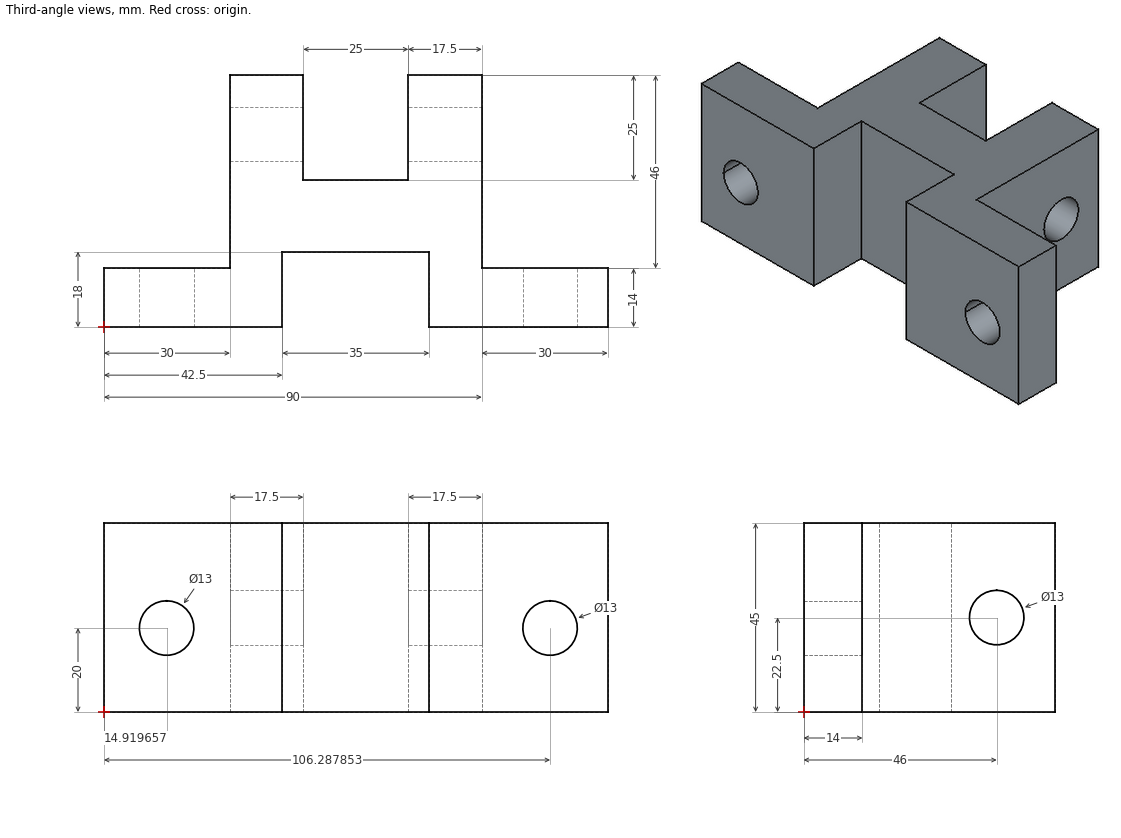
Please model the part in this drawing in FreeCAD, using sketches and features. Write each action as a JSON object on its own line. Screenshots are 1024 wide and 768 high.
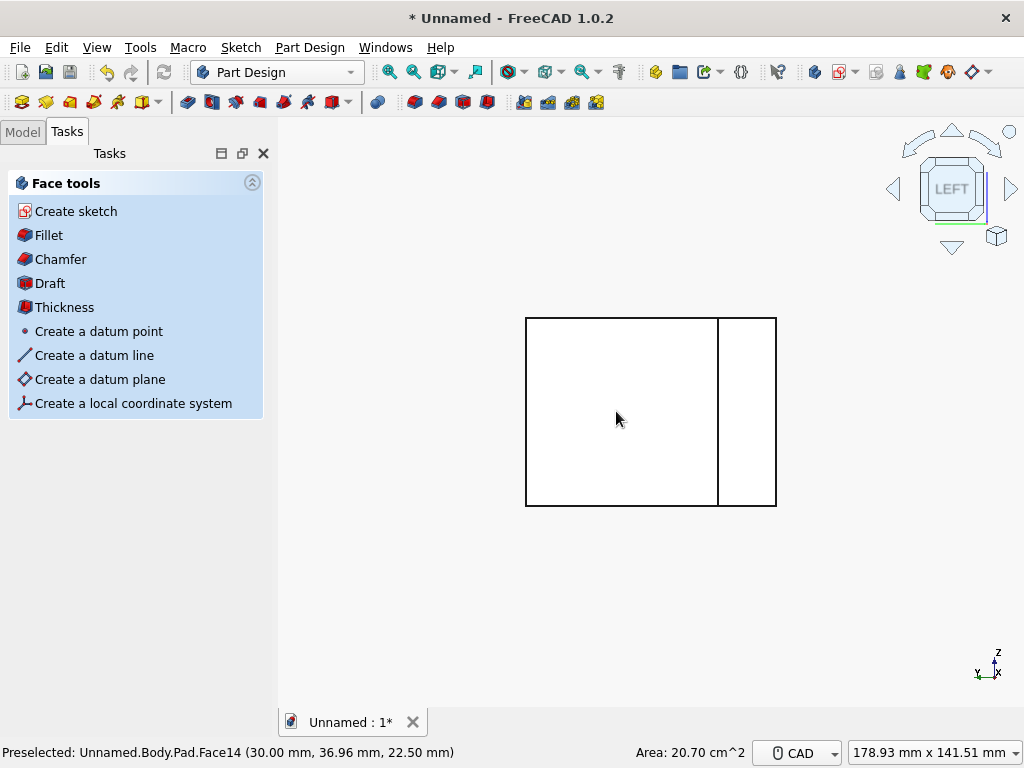
{"action": "left_click", "coordinate": [840, 72]}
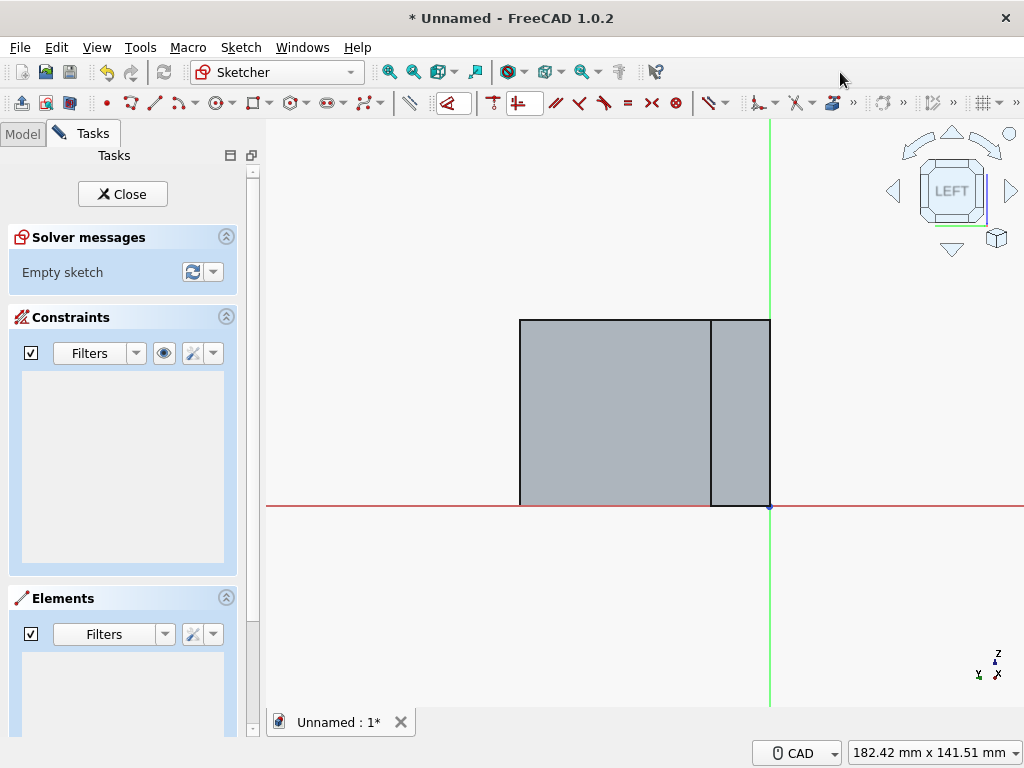
{"action": "scroll", "coordinate": [579, 413], "scroll_direction": "up", "scroll_amount": 10}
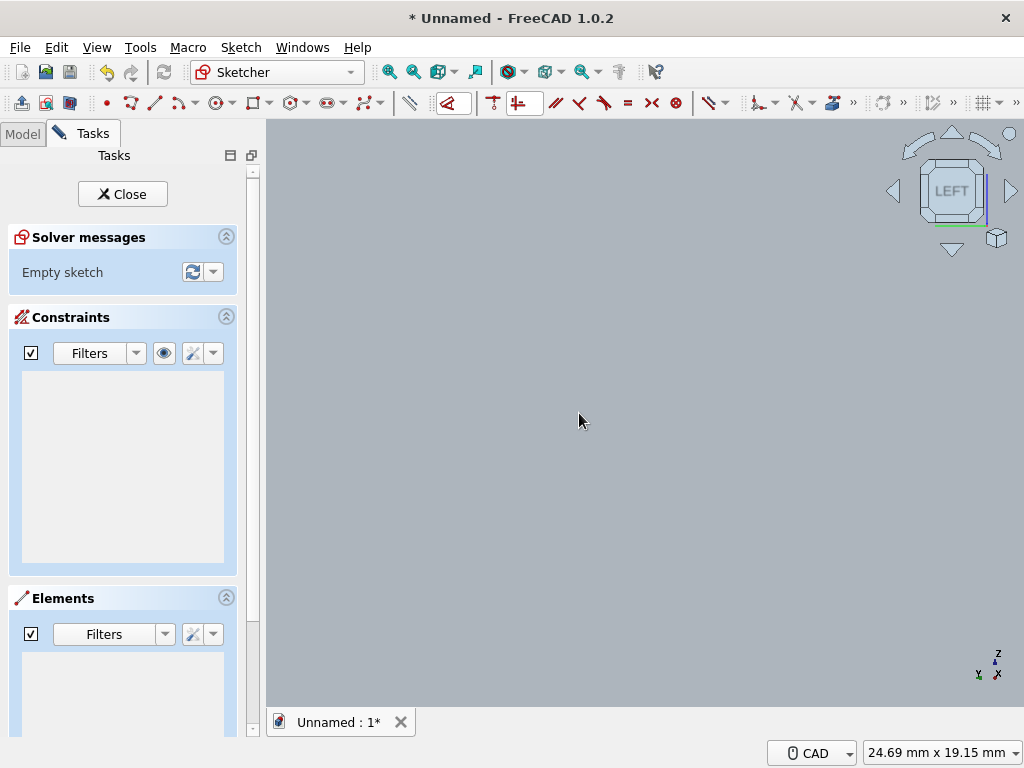
{"action": "left_click", "coordinate": [216, 104]}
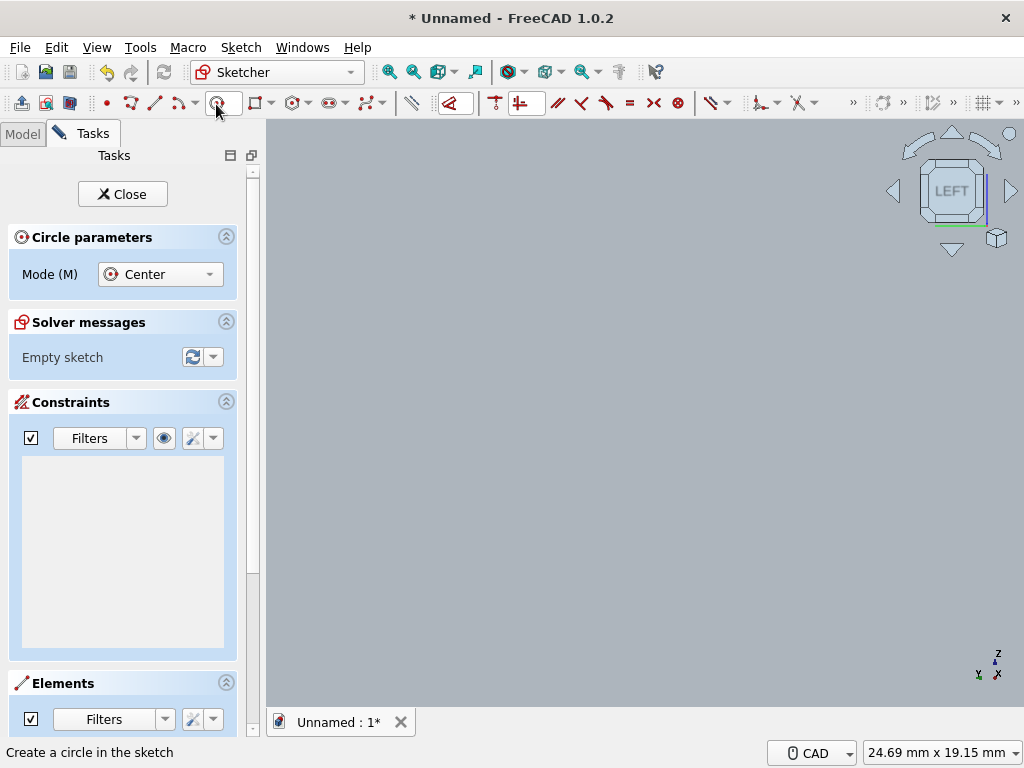
{"action": "left_click", "coordinate": [573, 410]}
{"action": "mouse_move", "coordinate": [714, 269]}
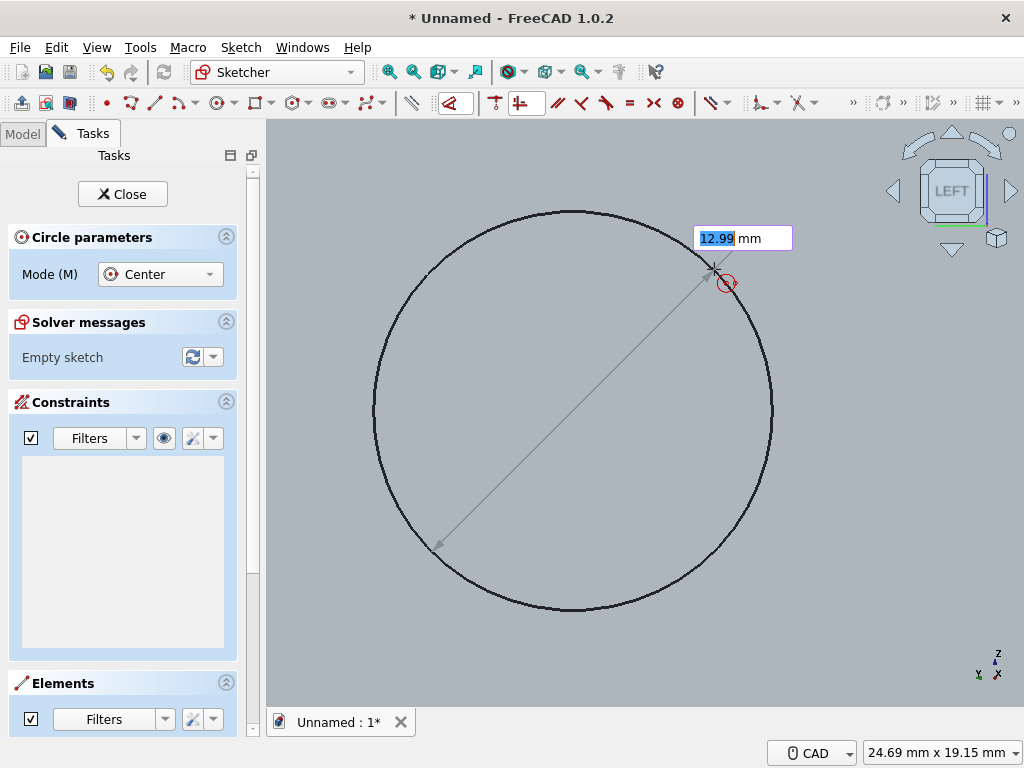
{"action": "type", "text": "13"}
{"action": "key", "text": "Return"}
{"action": "key", "text": "Escape"}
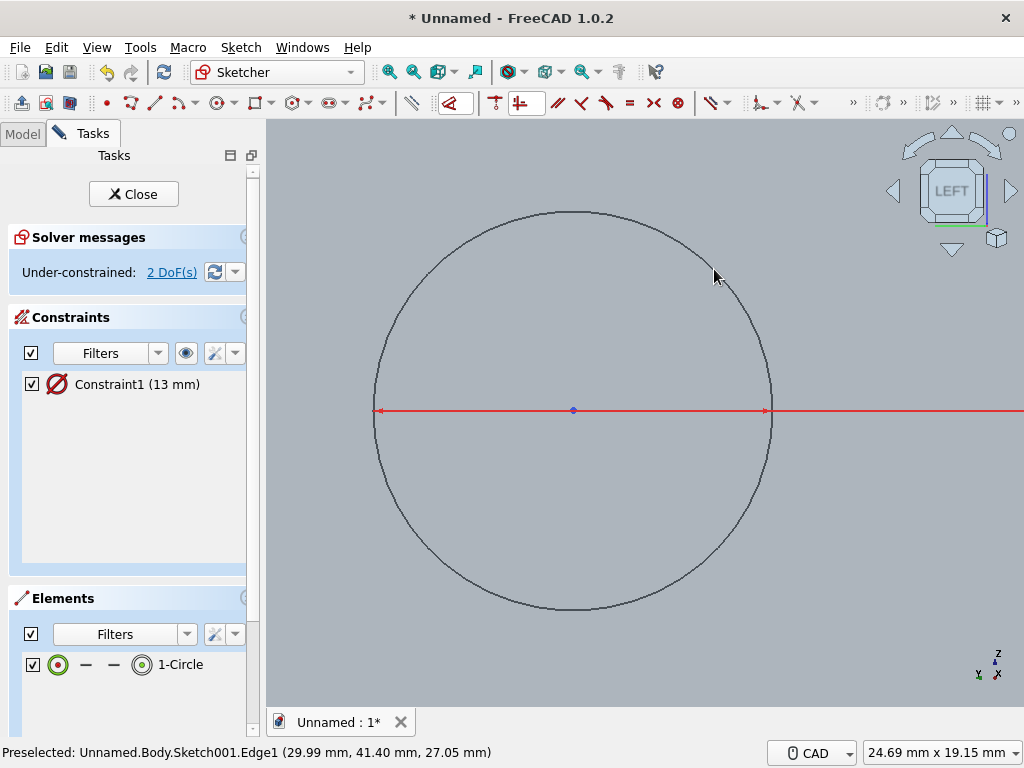
{"action": "left_click", "coordinate": [573, 411]}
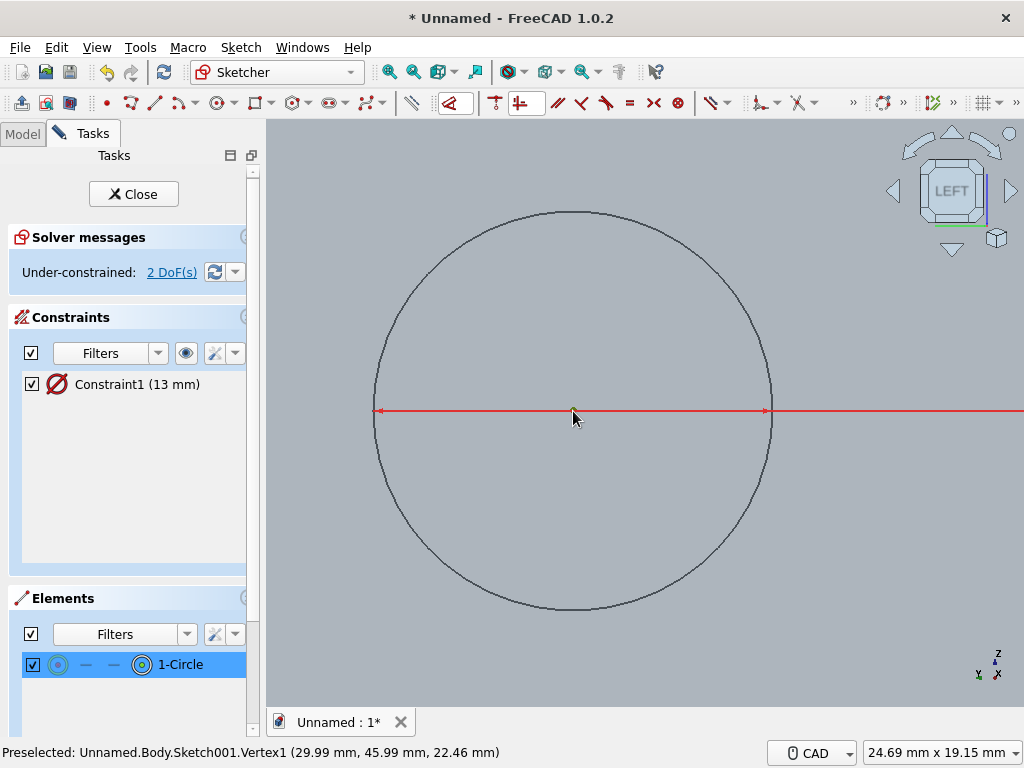
{"action": "key", "text": "l"}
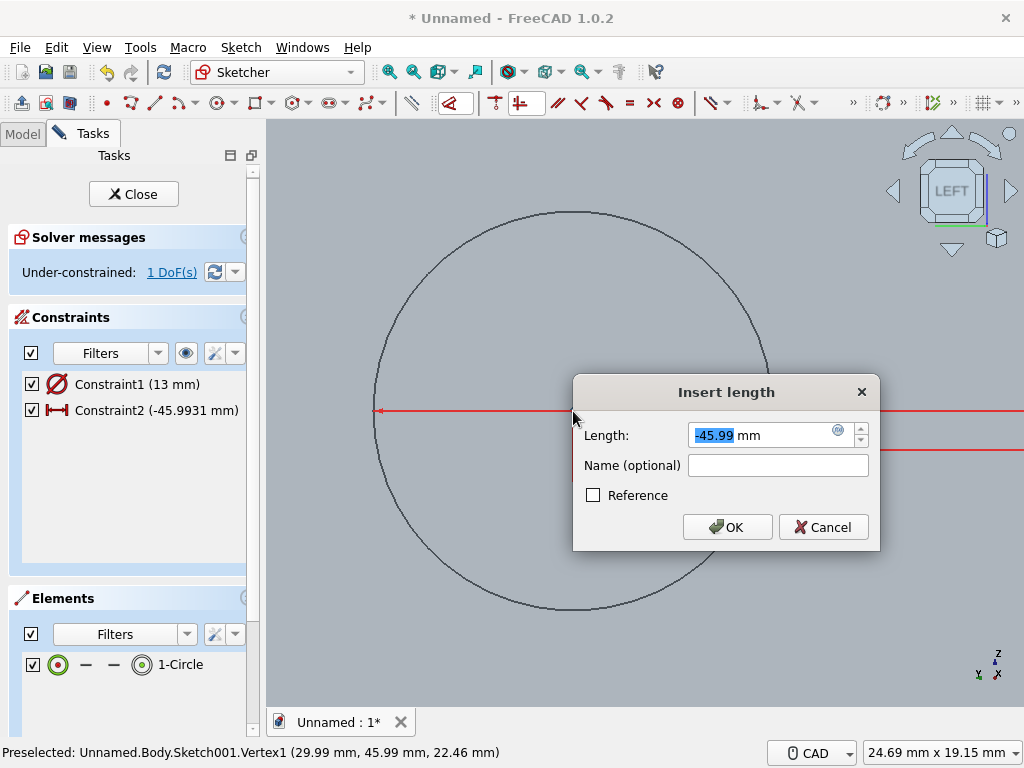
{"action": "type", "text": "-46"}
{"action": "key", "text": "Return"}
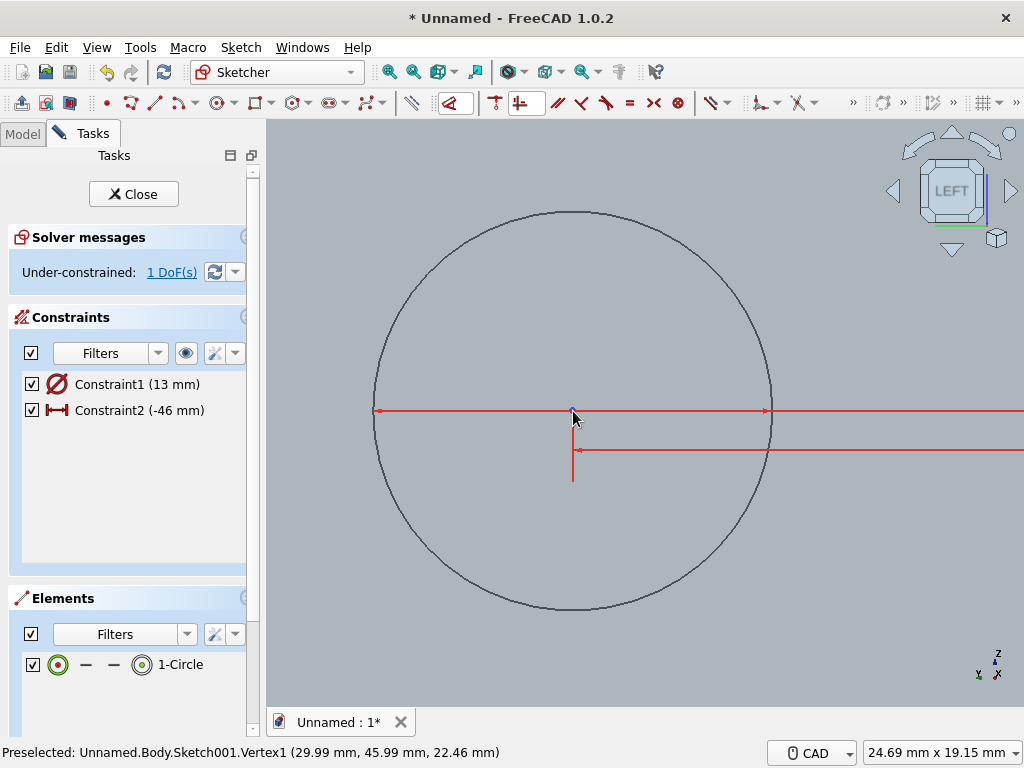
{"action": "left_click", "coordinate": [573, 411]}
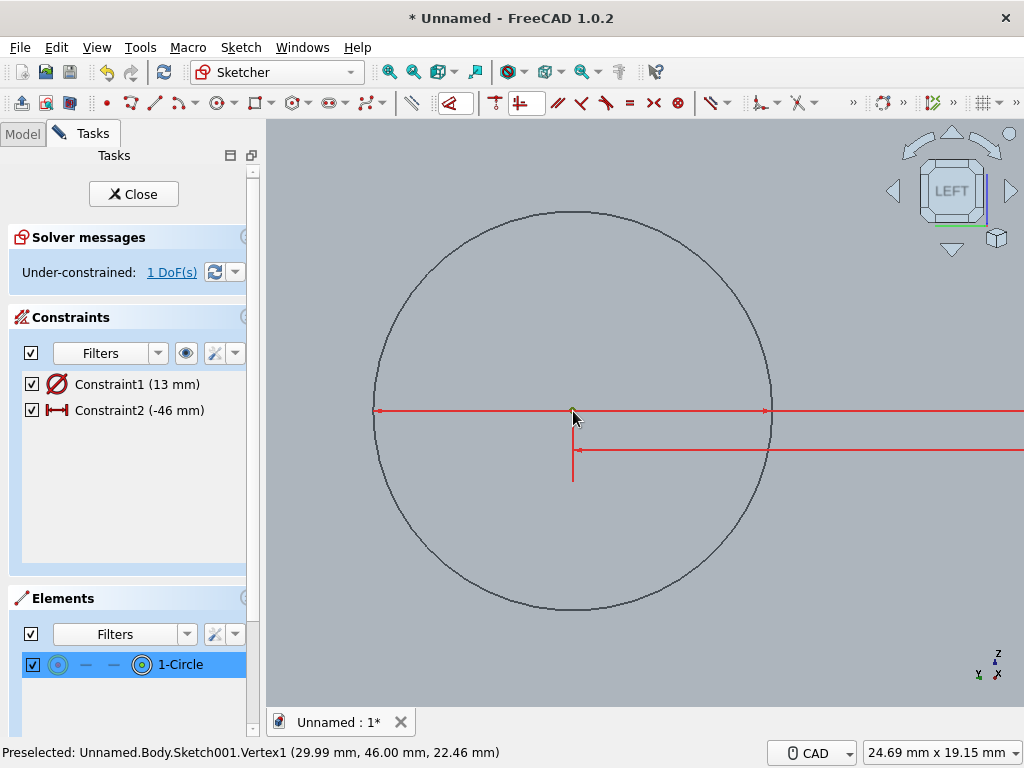
{"action": "key", "text": "i"}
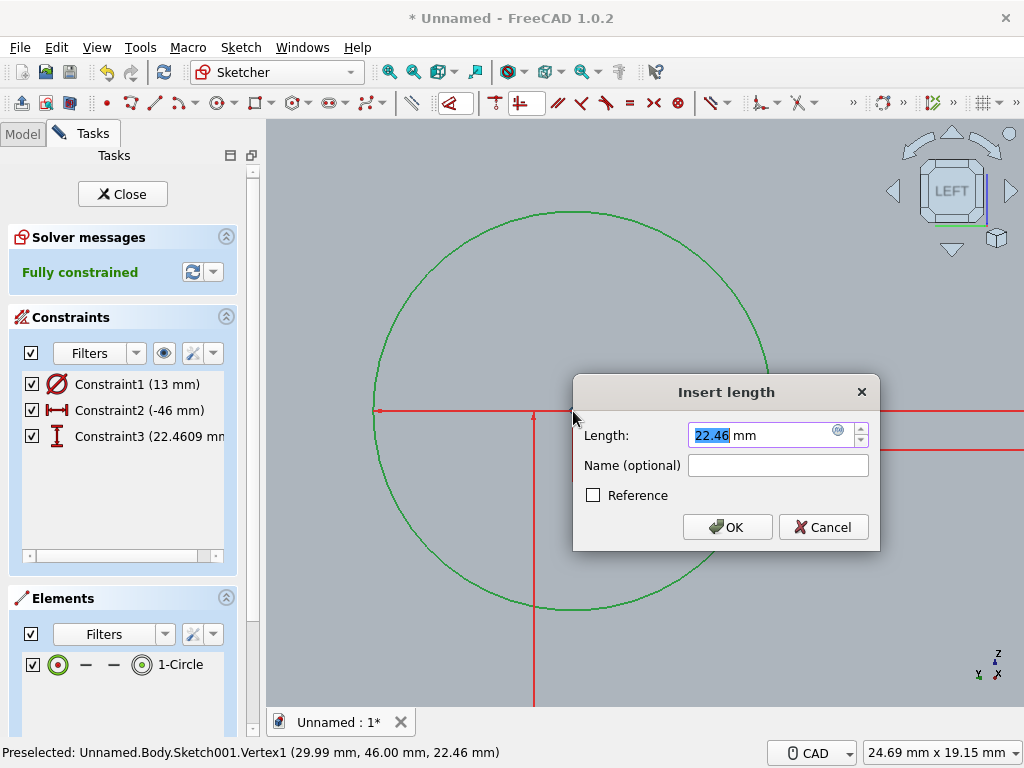
{"action": "type", "text": "22.5"}
{"action": "key", "text": "Return"}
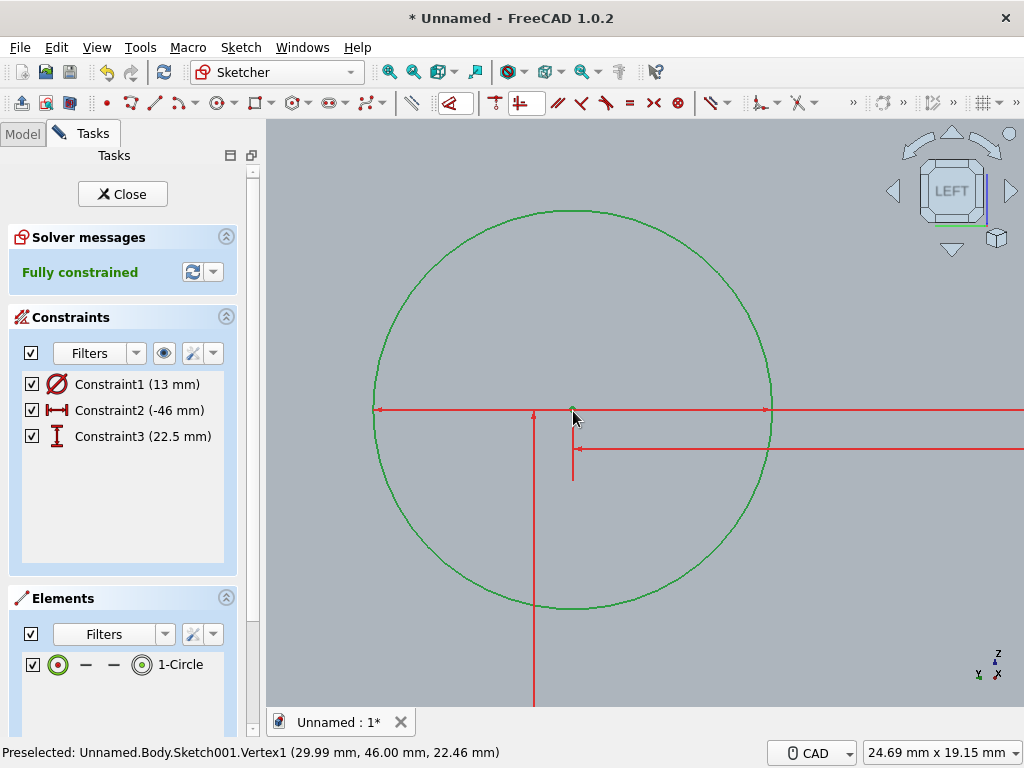
{"action": "left_click", "coordinate": [123, 194]}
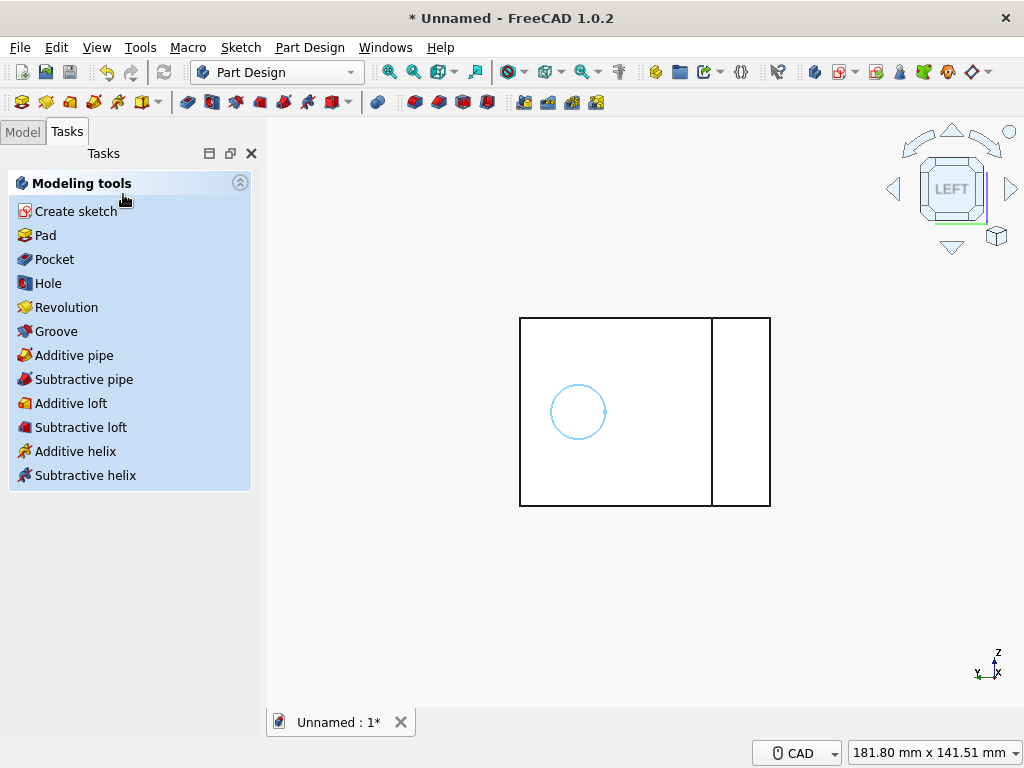
{"action": "left_click", "coordinate": [188, 102]}